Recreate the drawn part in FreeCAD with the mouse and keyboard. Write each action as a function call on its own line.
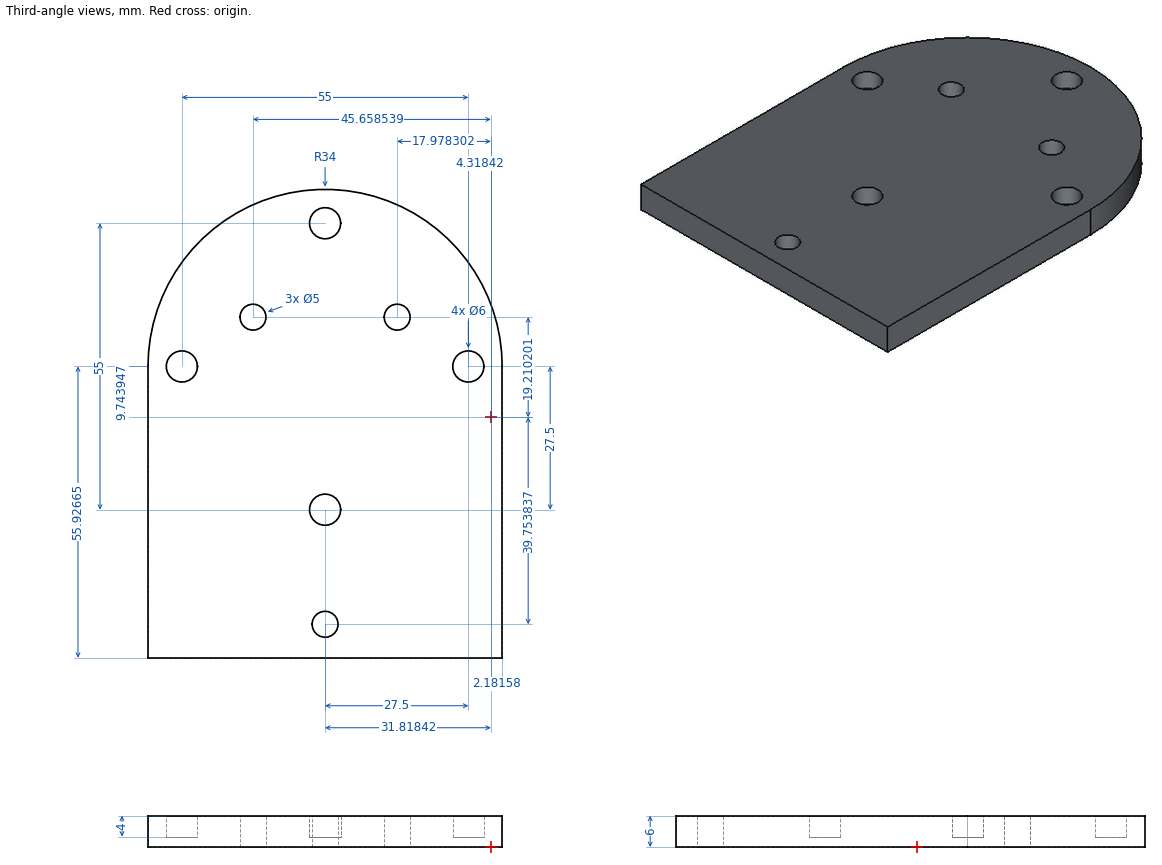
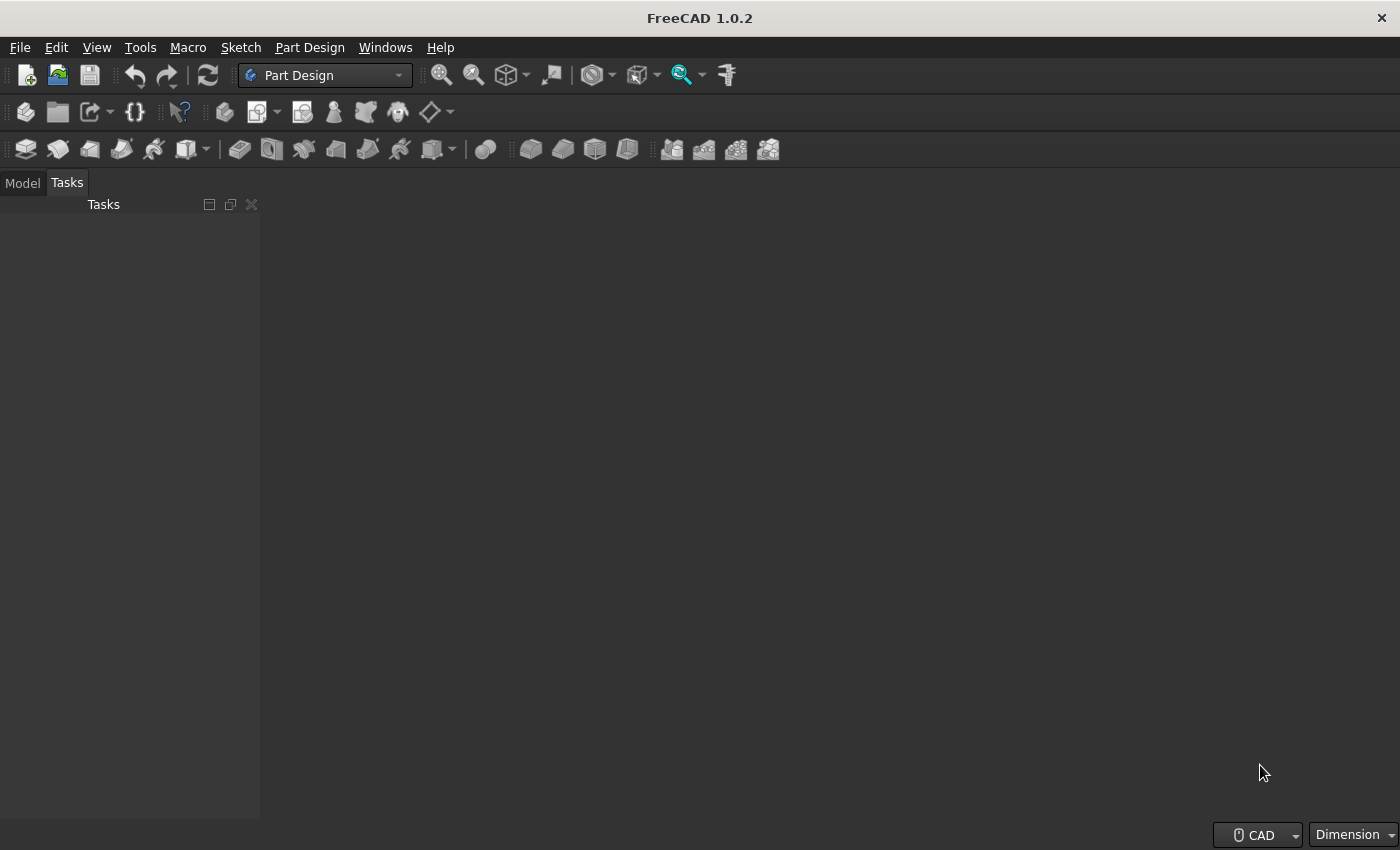
click(26, 76)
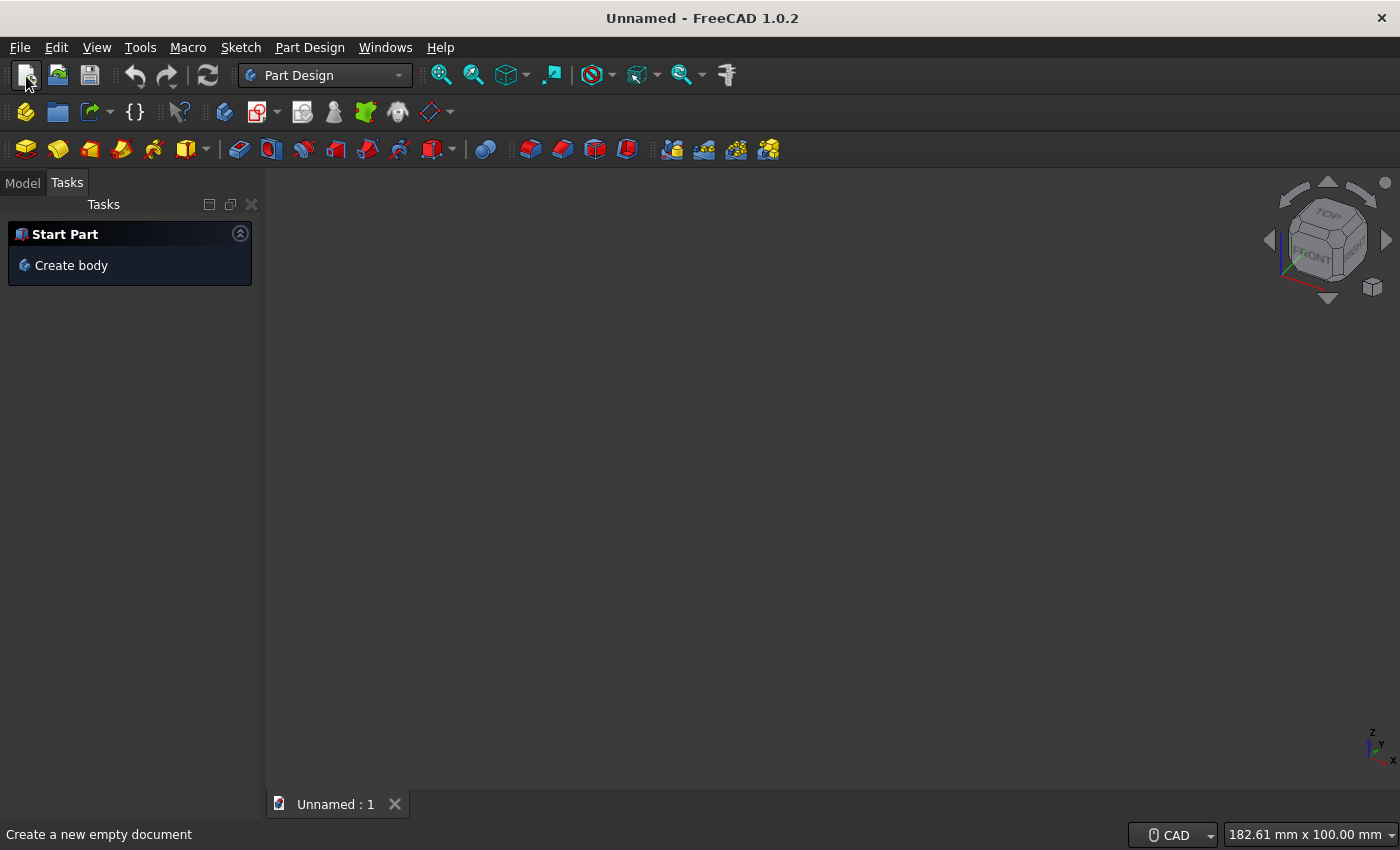
click(258, 112)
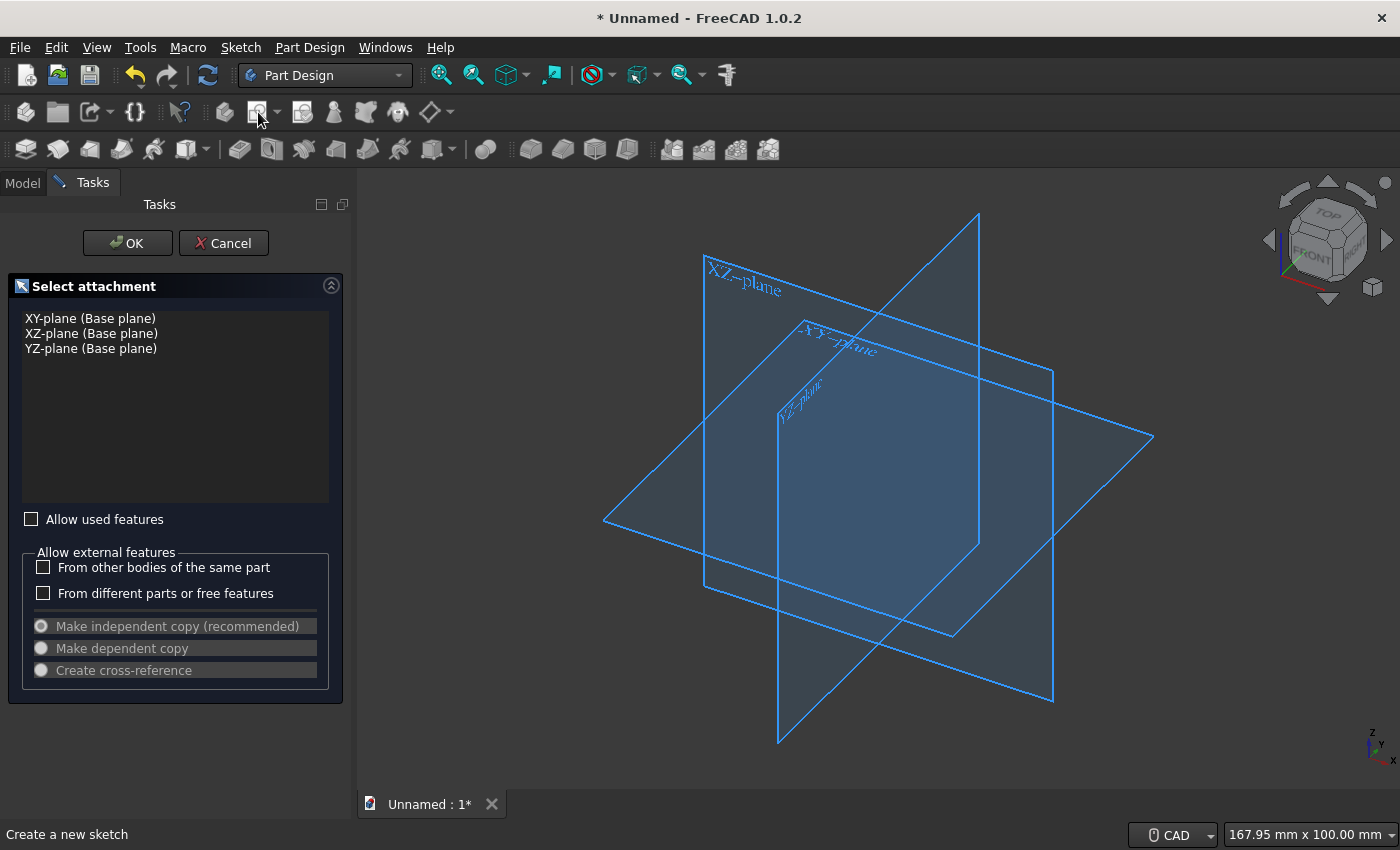
click(82, 318)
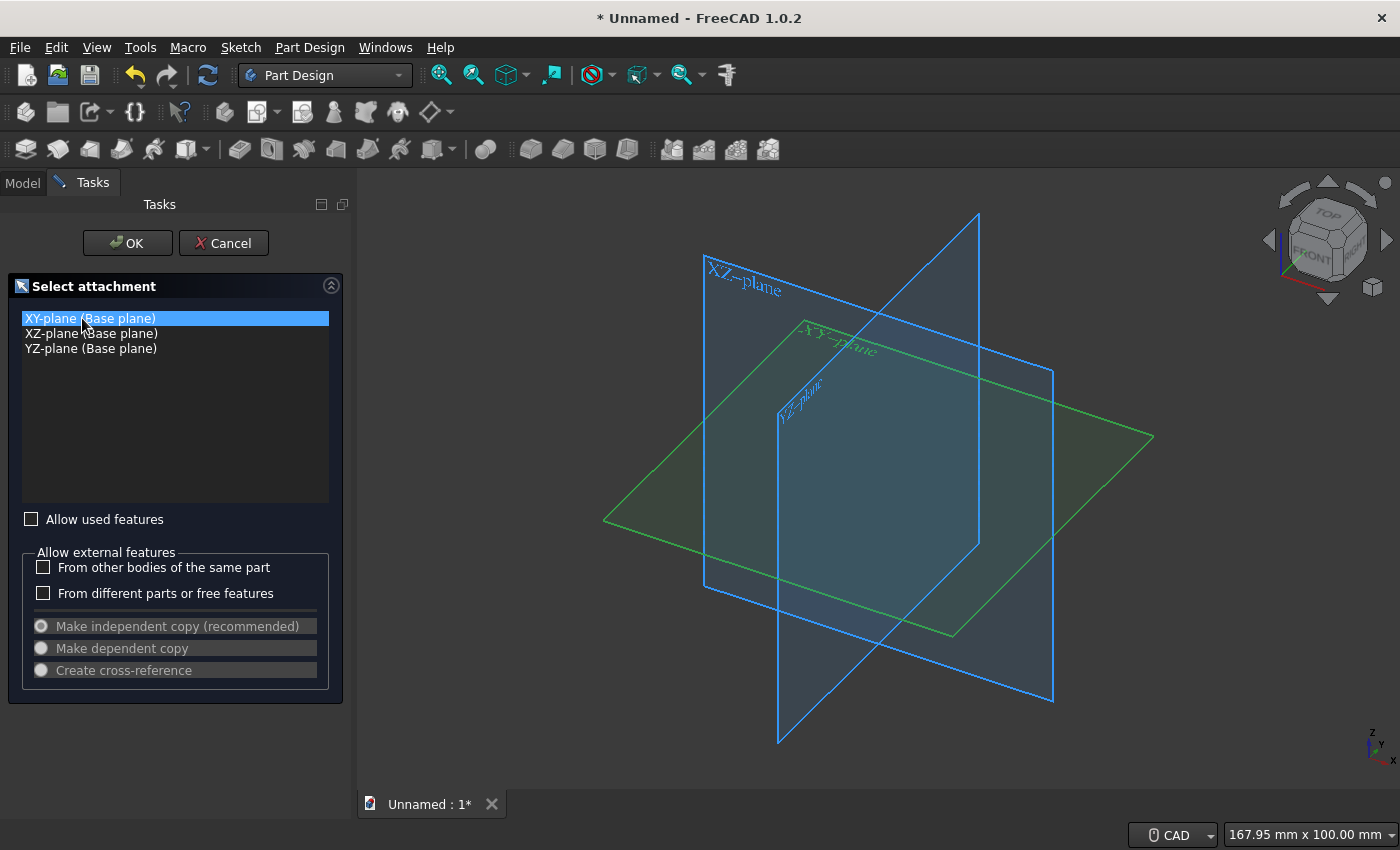
click(128, 243)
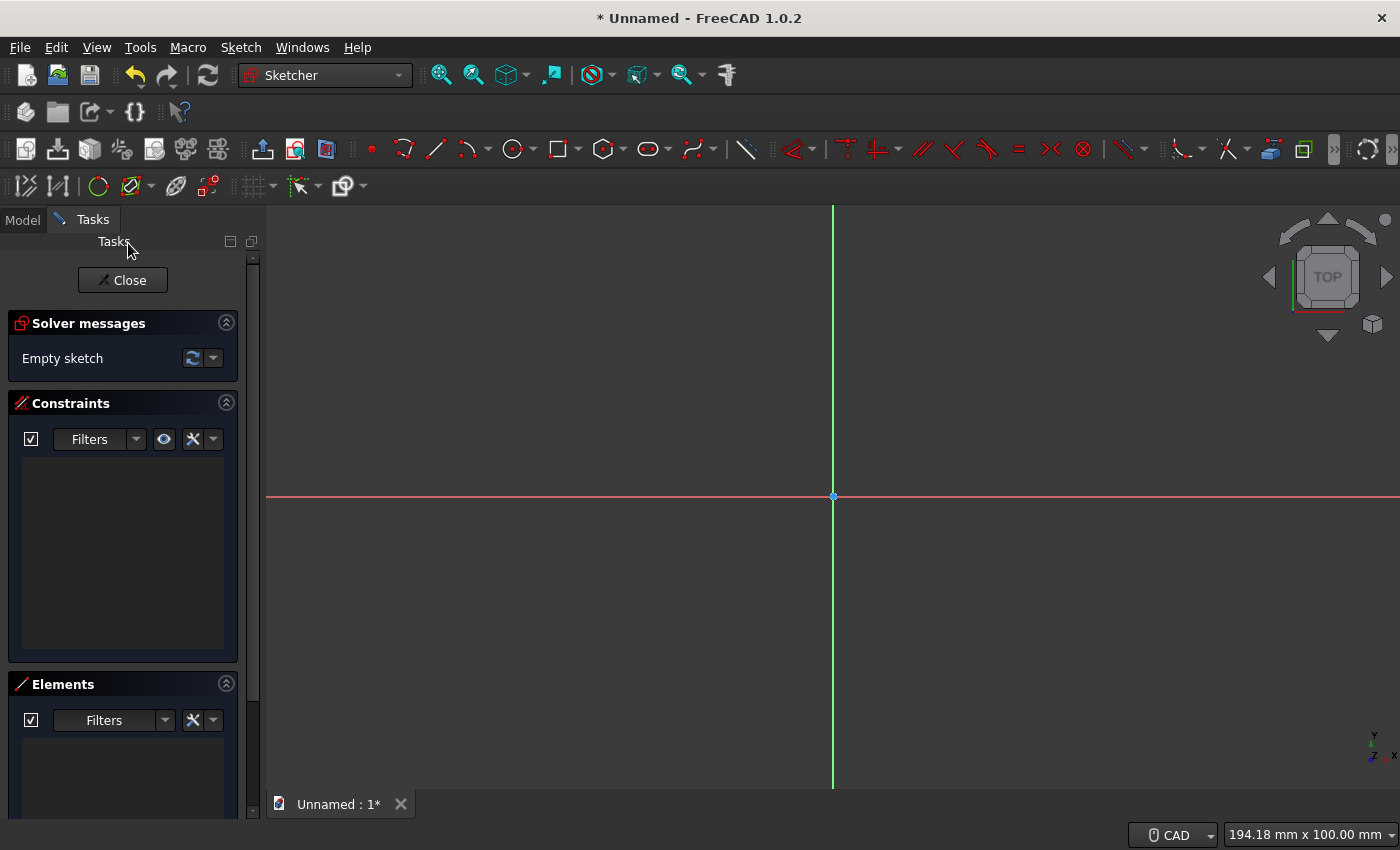
scroll(1003, 483, down, 2)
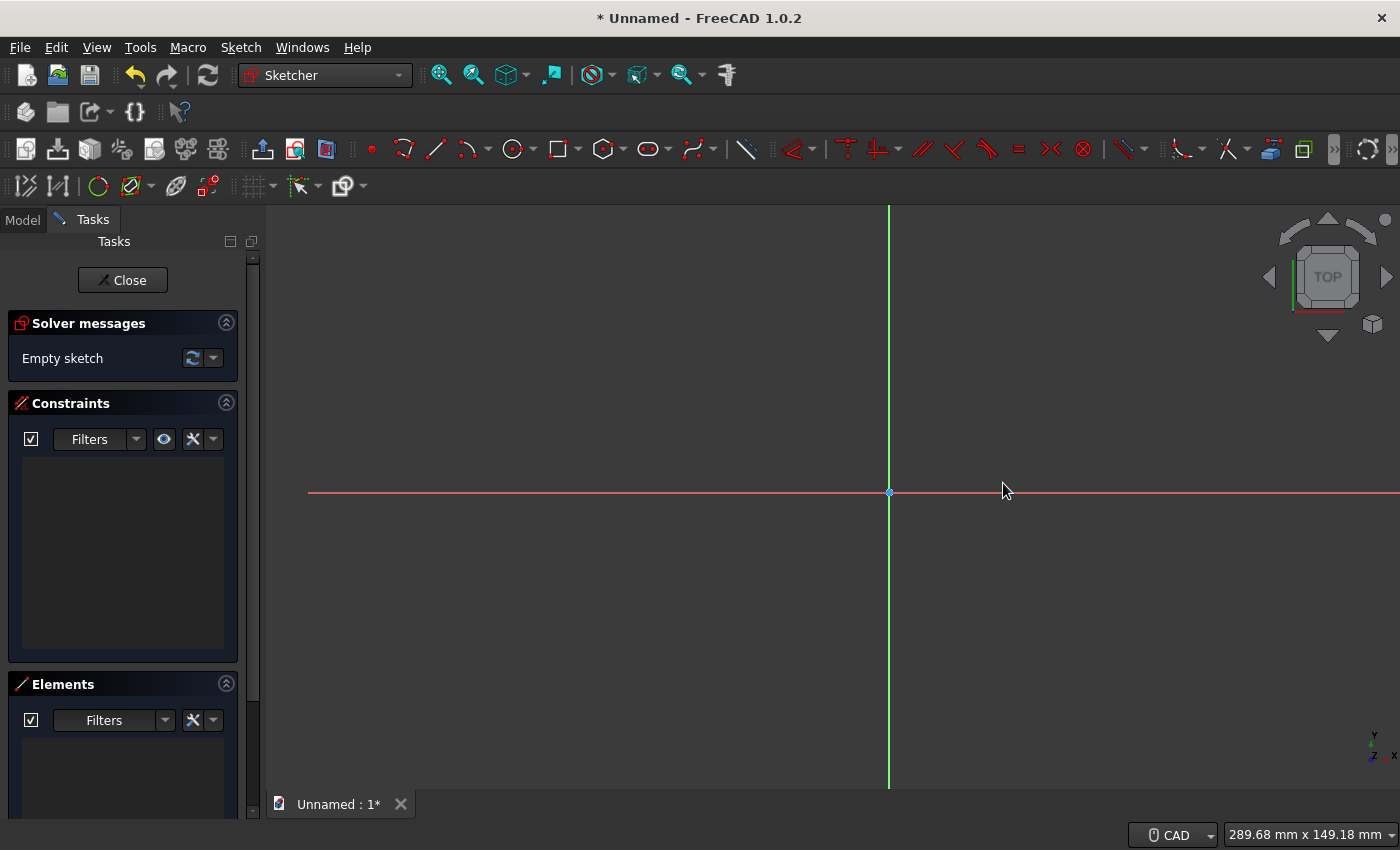
key(g)
key(m)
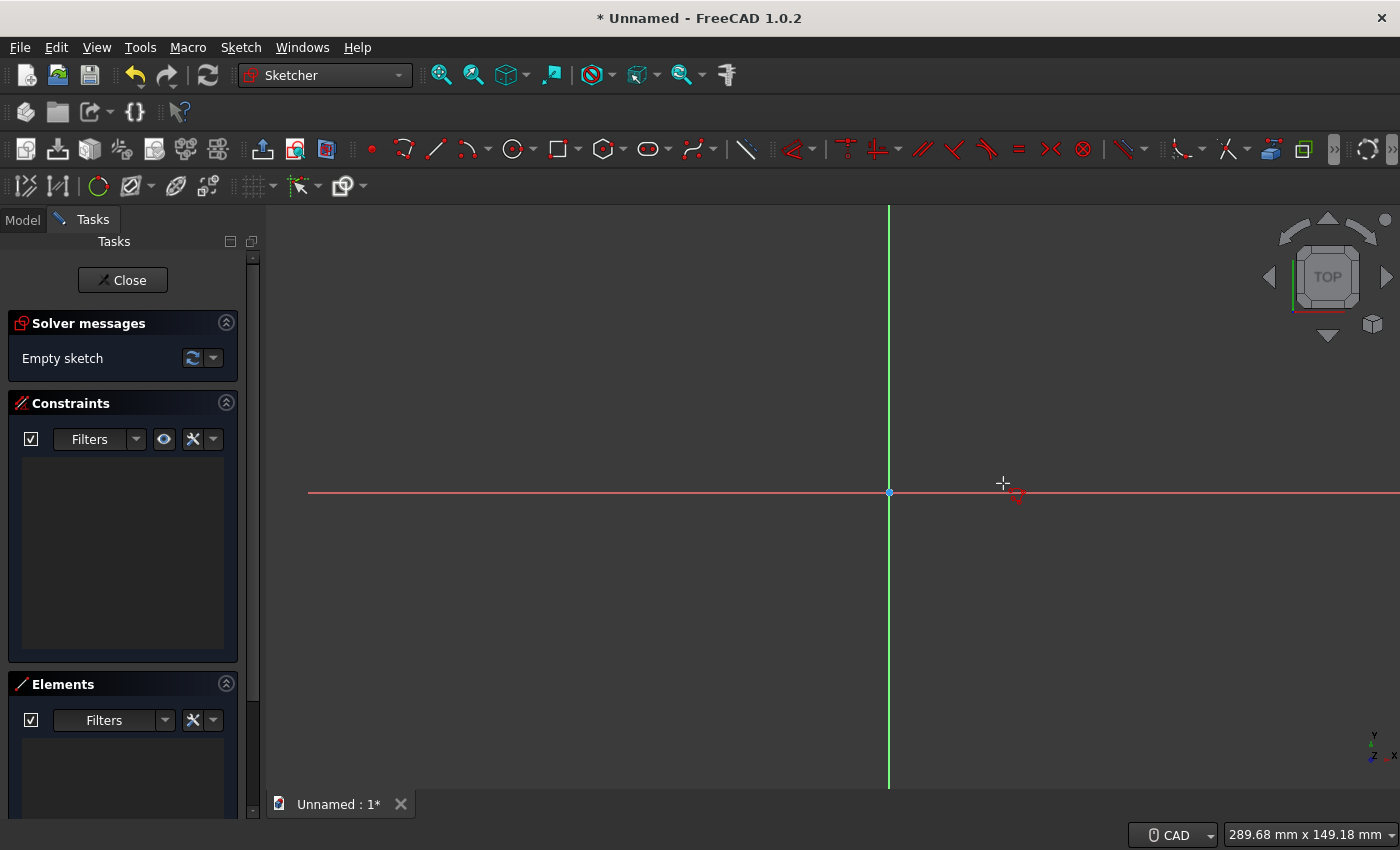
click(632, 454)
click(632, 673)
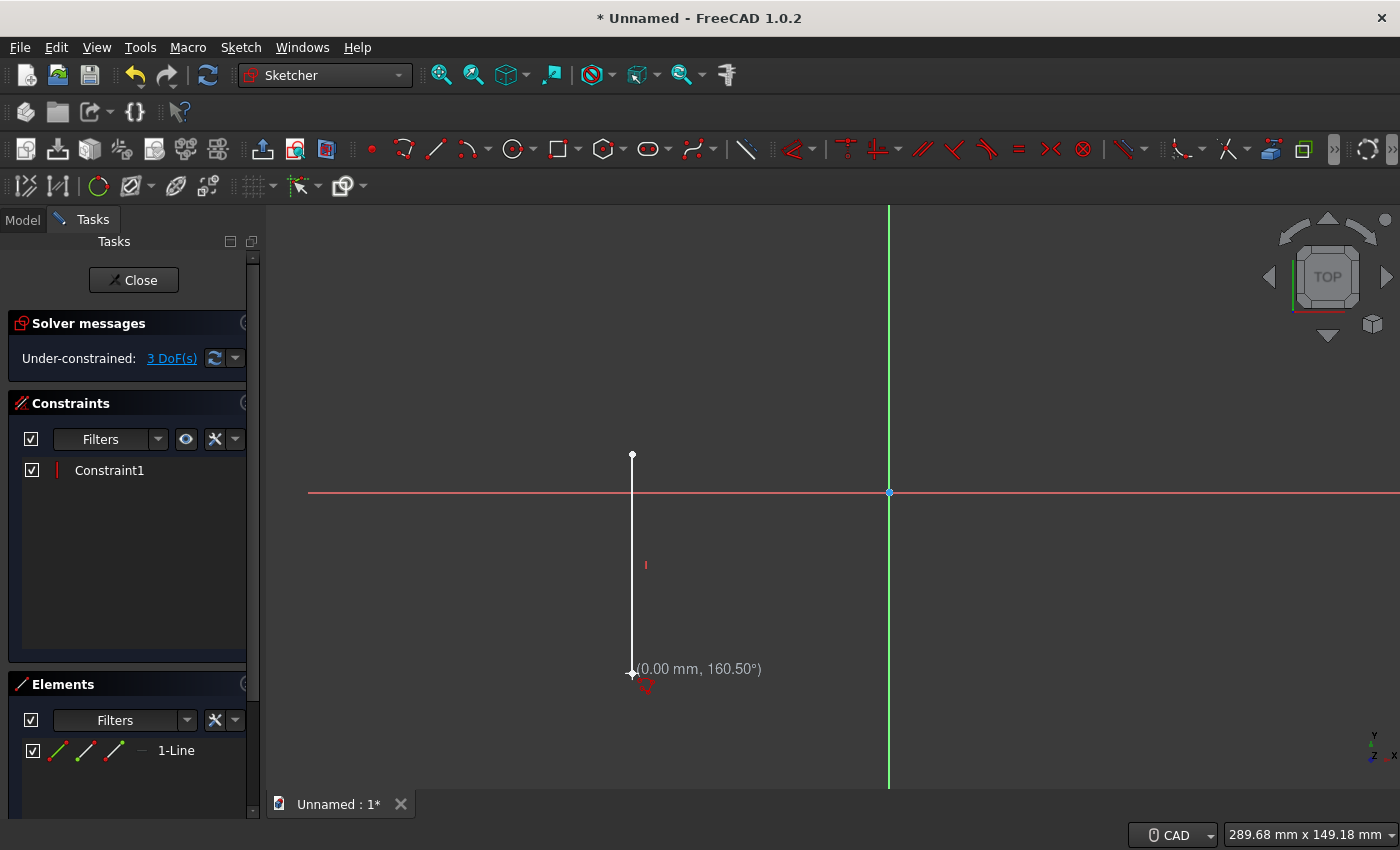
scroll(898, 673, up, 4)